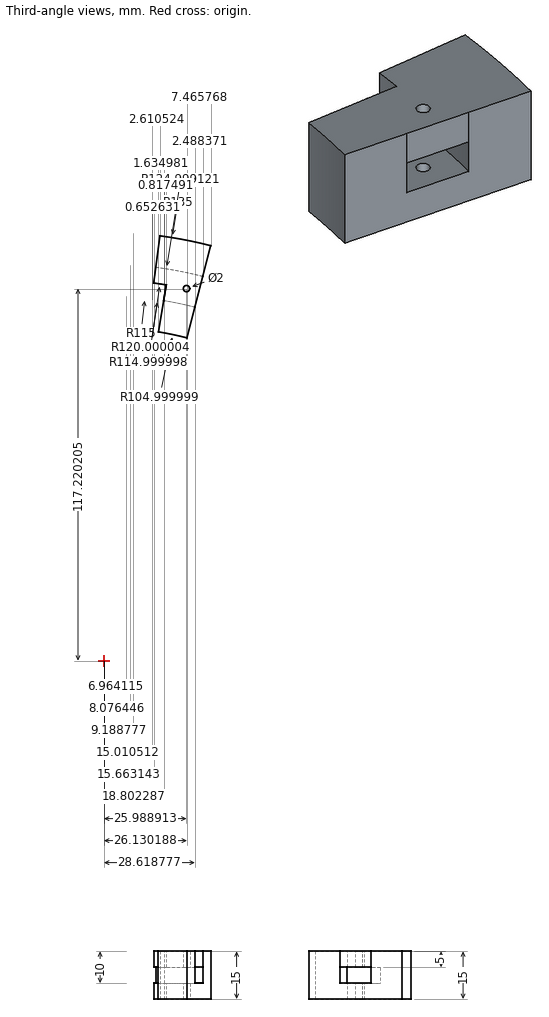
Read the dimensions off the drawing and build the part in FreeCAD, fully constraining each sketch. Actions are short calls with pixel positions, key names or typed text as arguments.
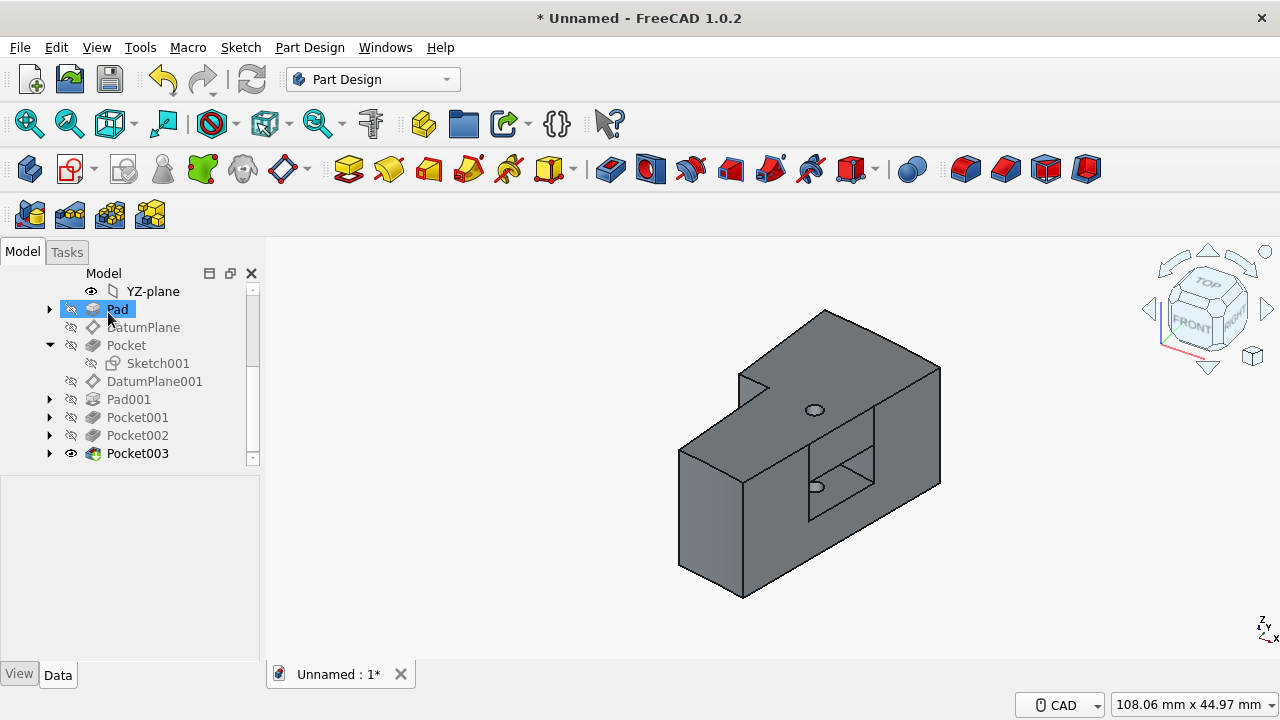
key(0)